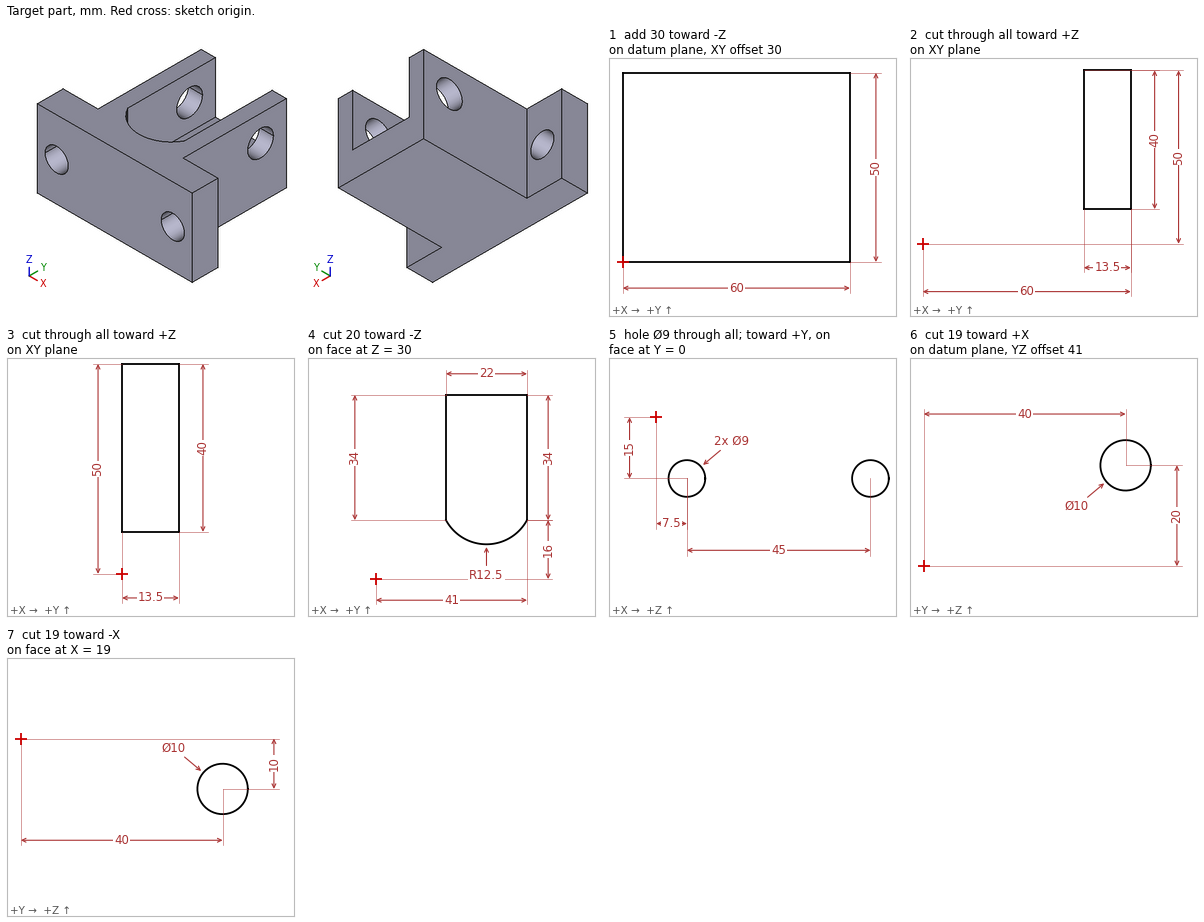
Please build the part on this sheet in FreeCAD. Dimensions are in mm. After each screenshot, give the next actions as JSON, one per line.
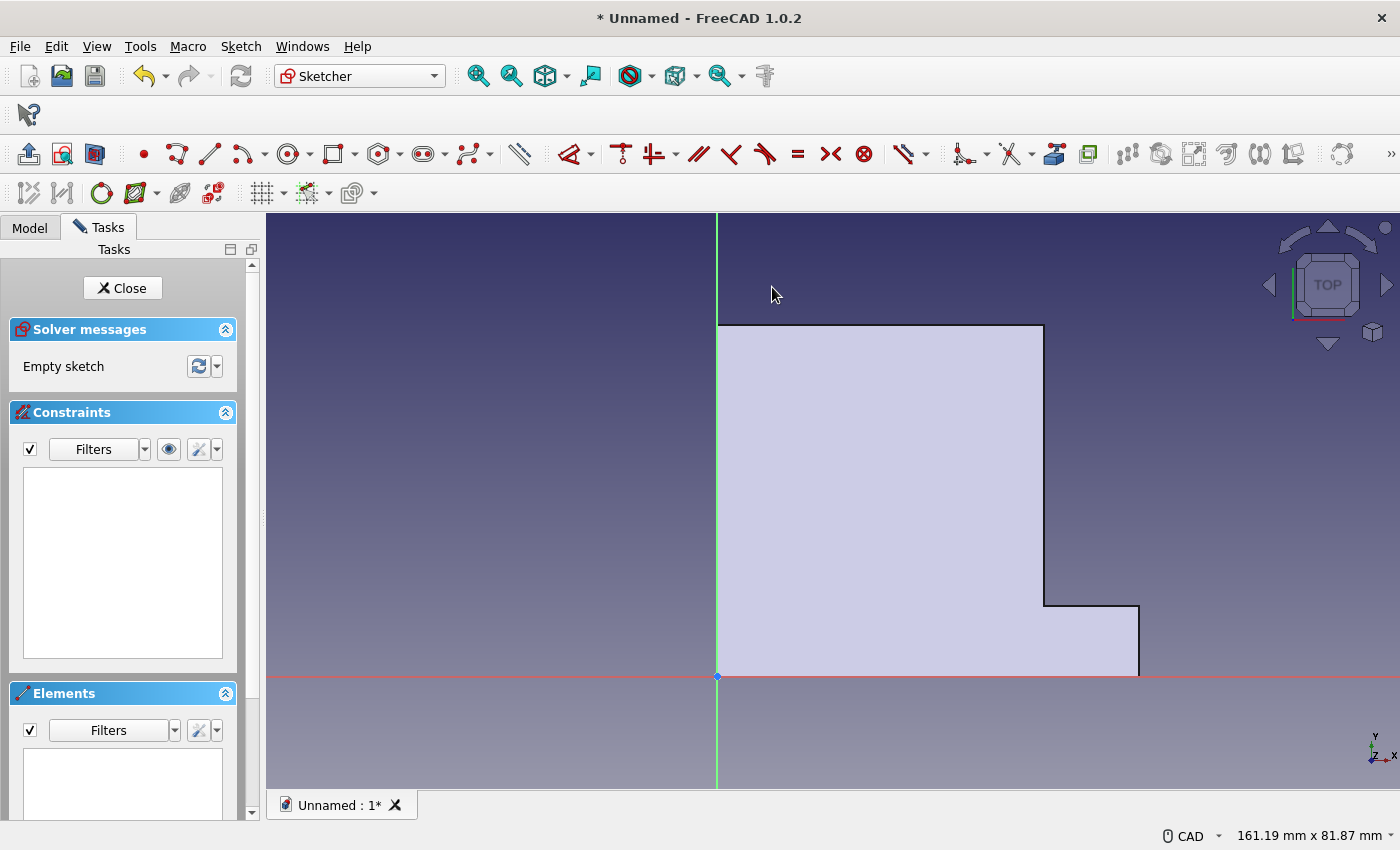
{"action": "left_click", "coordinate": [332, 154]}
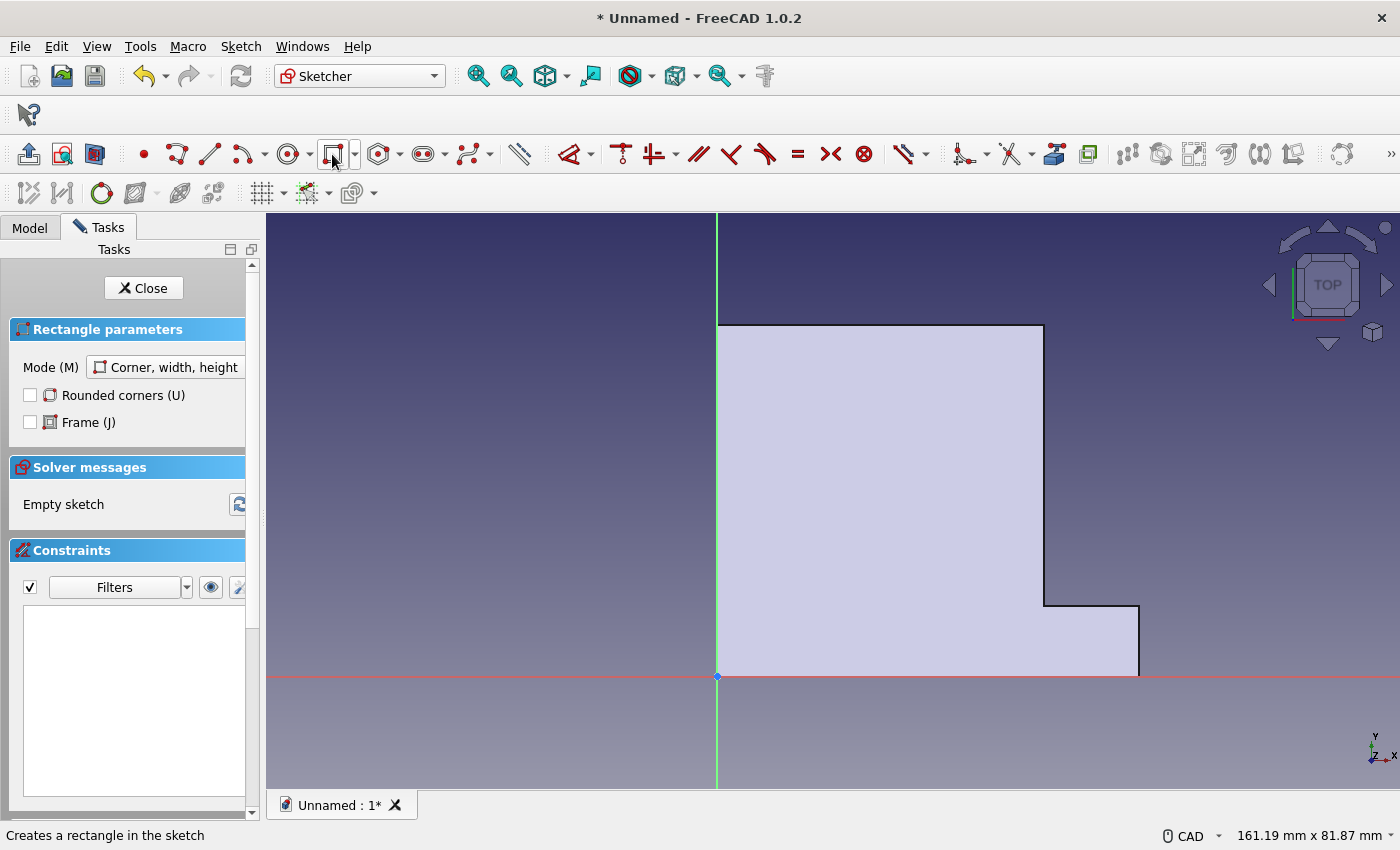
{"action": "left_click", "coordinate": [717, 325]}
{"action": "mouse_move", "coordinate": [812, 606]}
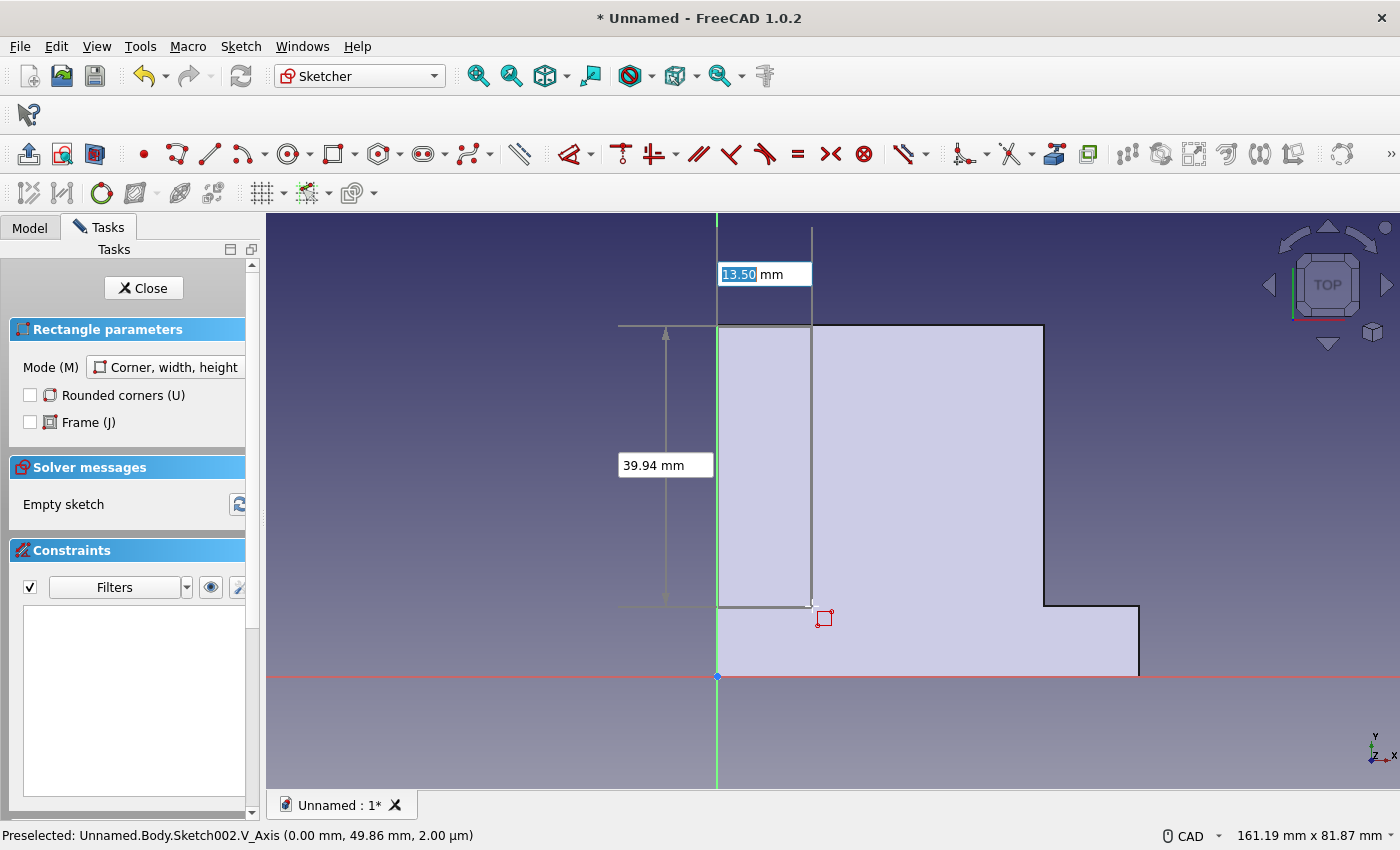
{"action": "type", "text": "13.5"}
{"action": "key", "text": "Tab"}
{"action": "type", "text": "40"}
{"action": "key", "text": "Return"}
{"action": "key", "text": "Escape"}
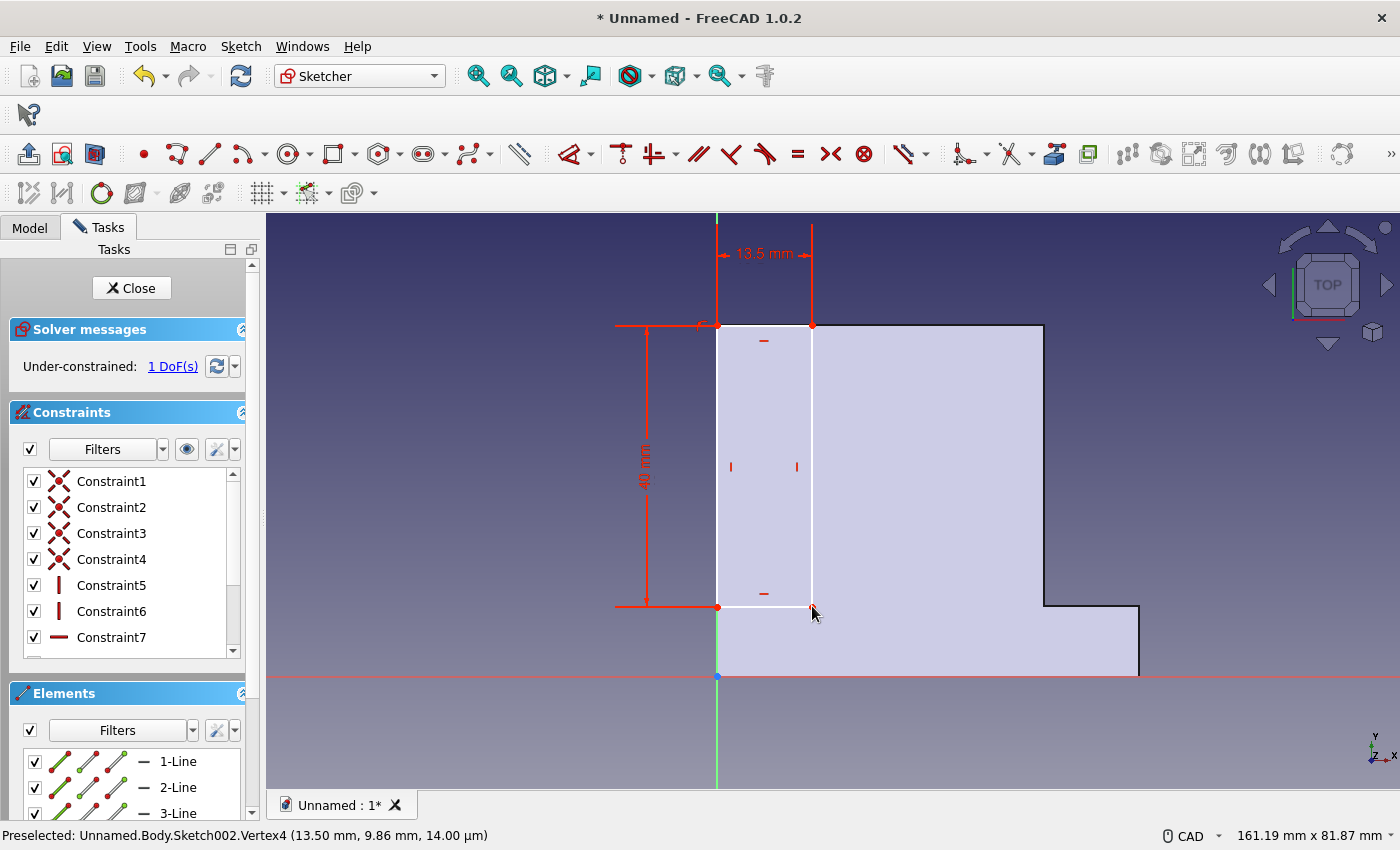
{"action": "left_click", "coordinate": [717, 326]}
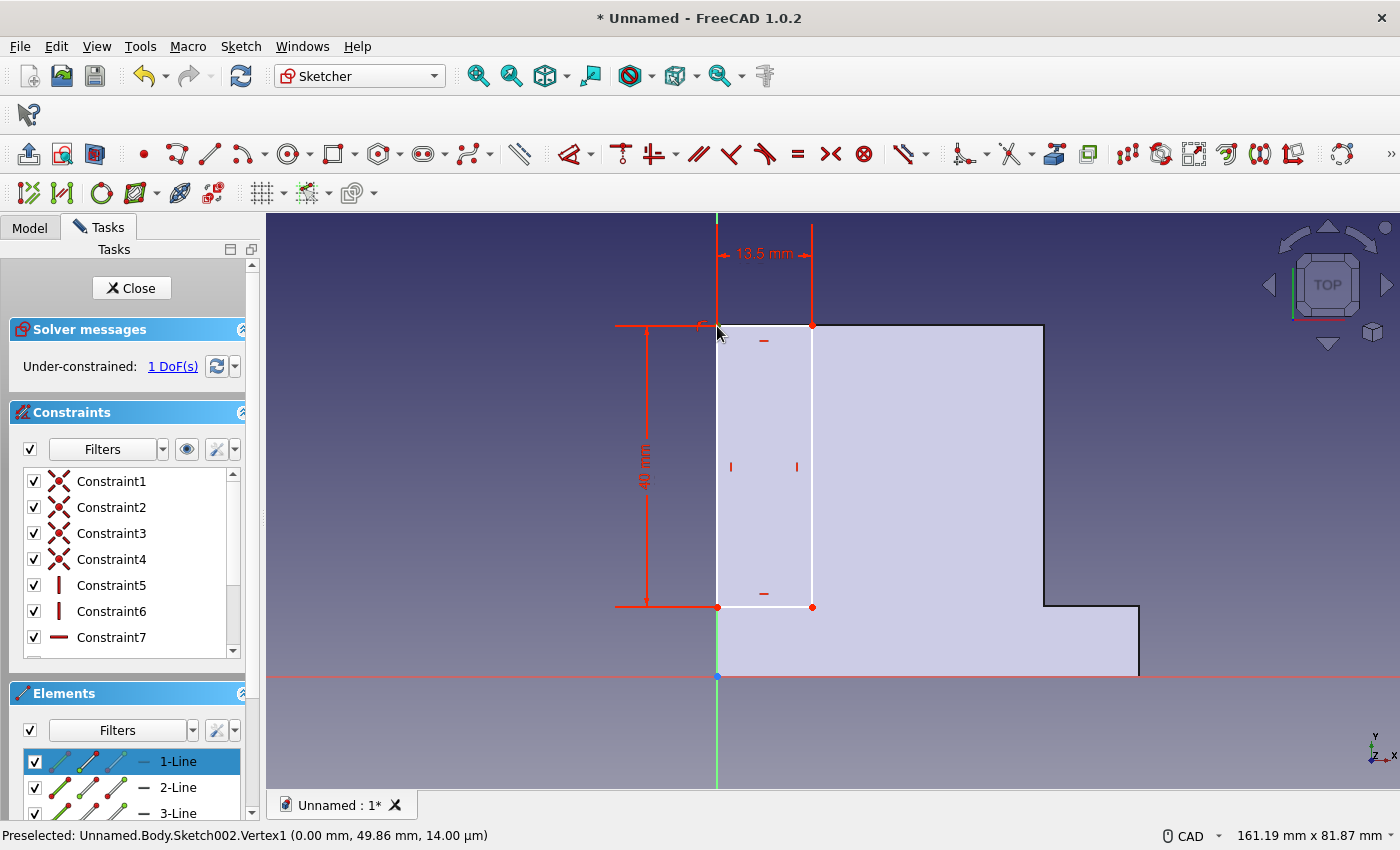
{"action": "key", "text": "i"}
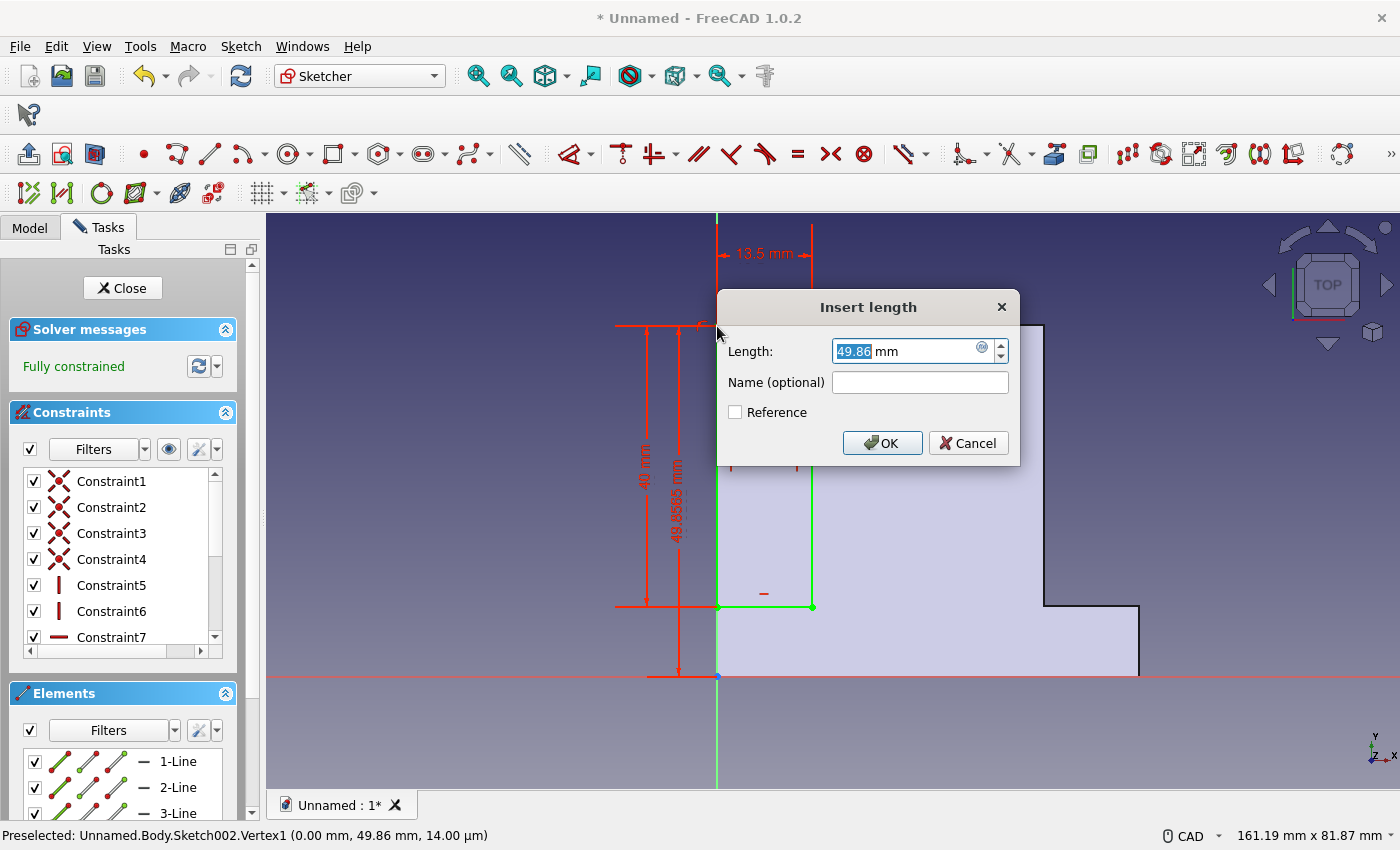
{"action": "type", "text": "50"}
{"action": "key", "text": "Return"}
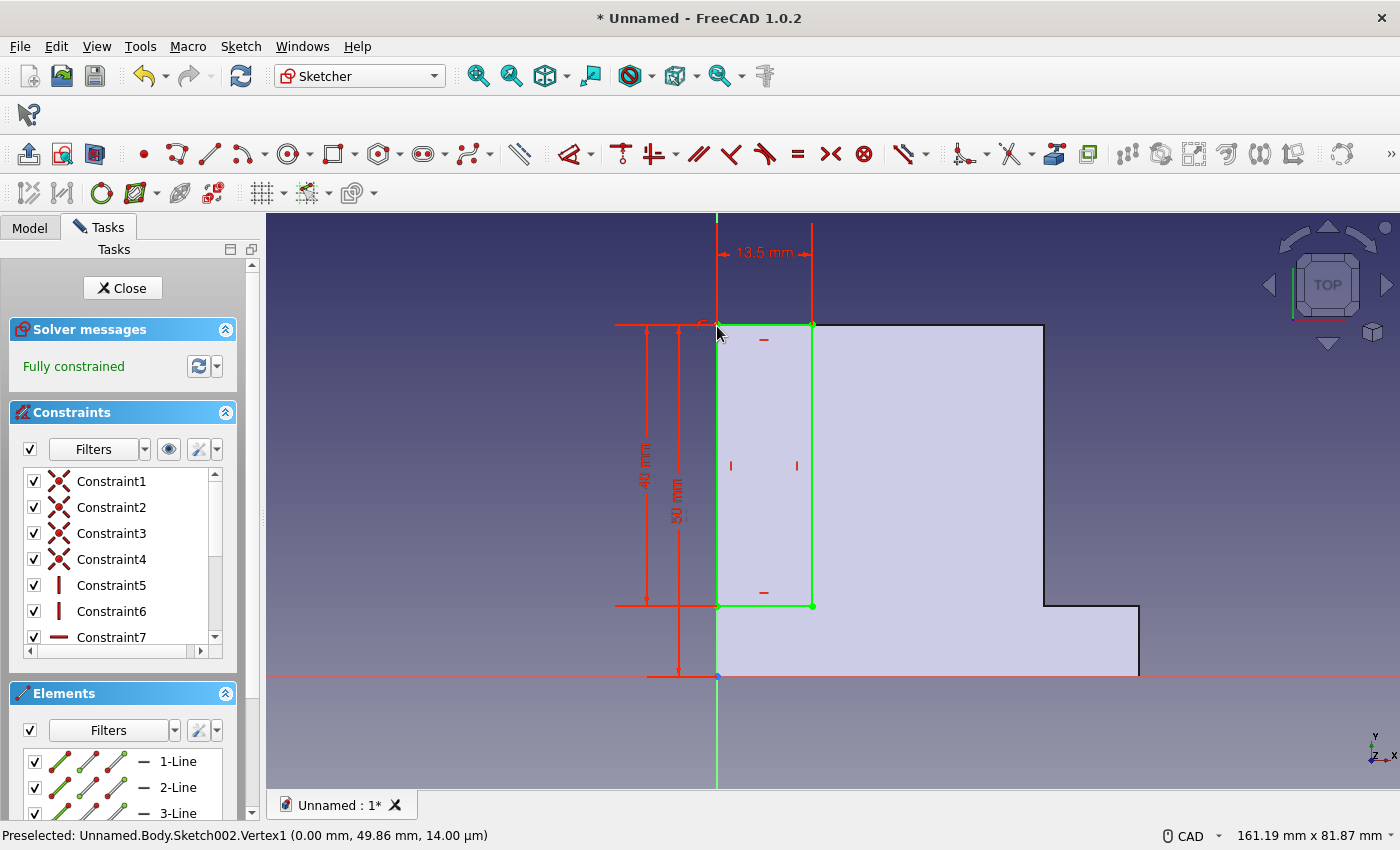
{"action": "left_click", "coordinate": [123, 288]}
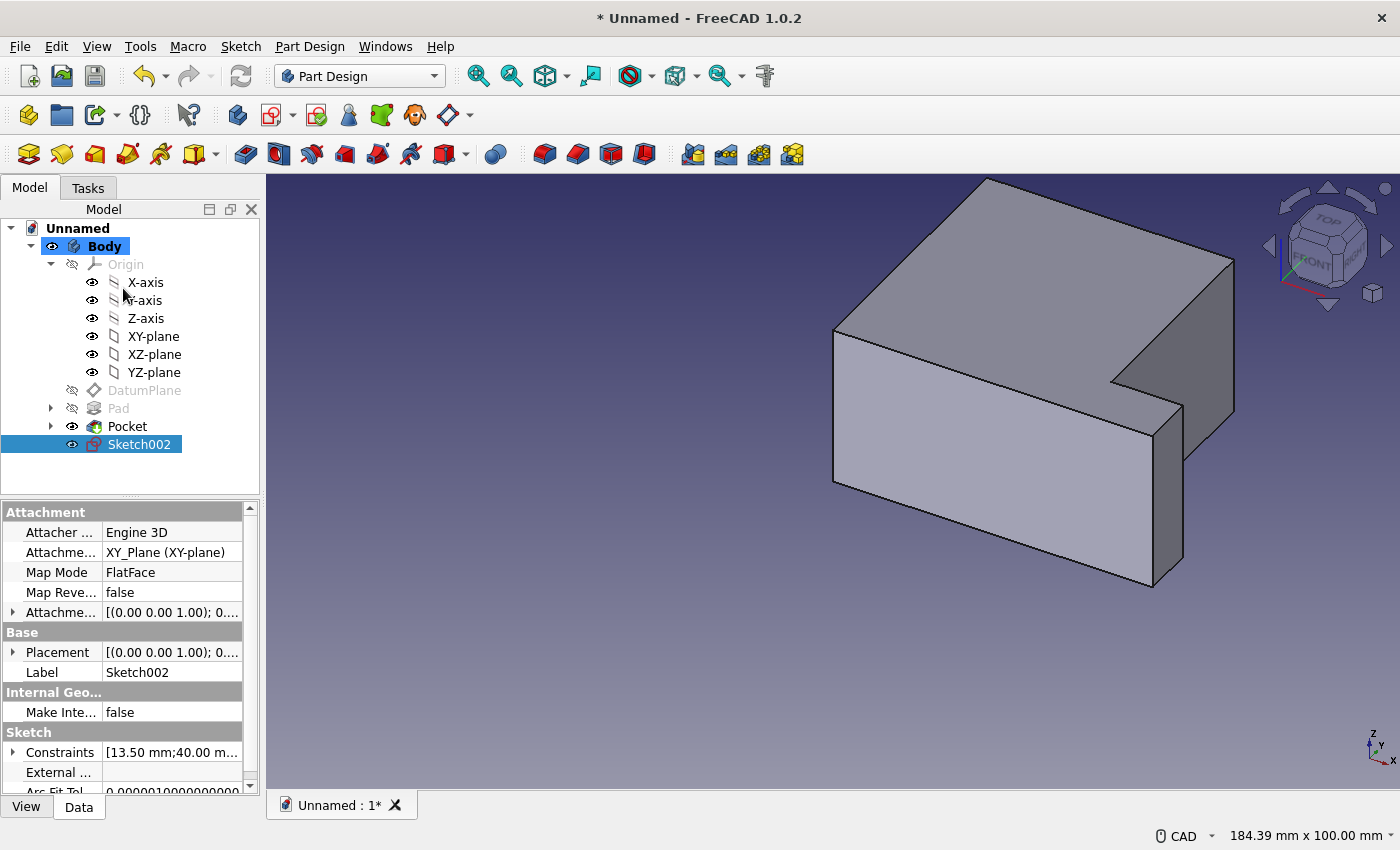
{"action": "left_click", "coordinate": [246, 154]}